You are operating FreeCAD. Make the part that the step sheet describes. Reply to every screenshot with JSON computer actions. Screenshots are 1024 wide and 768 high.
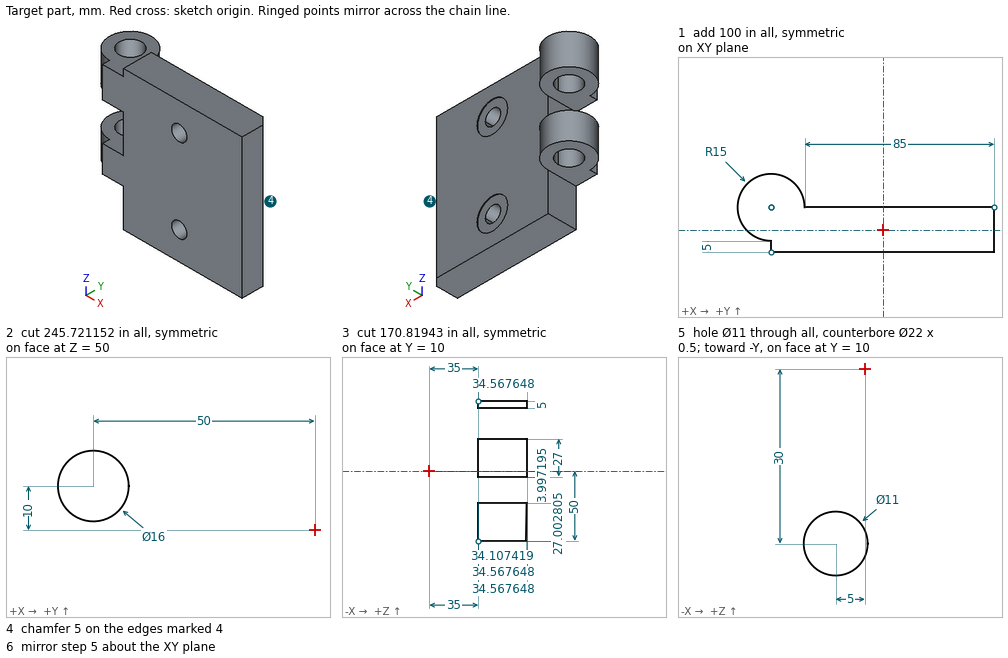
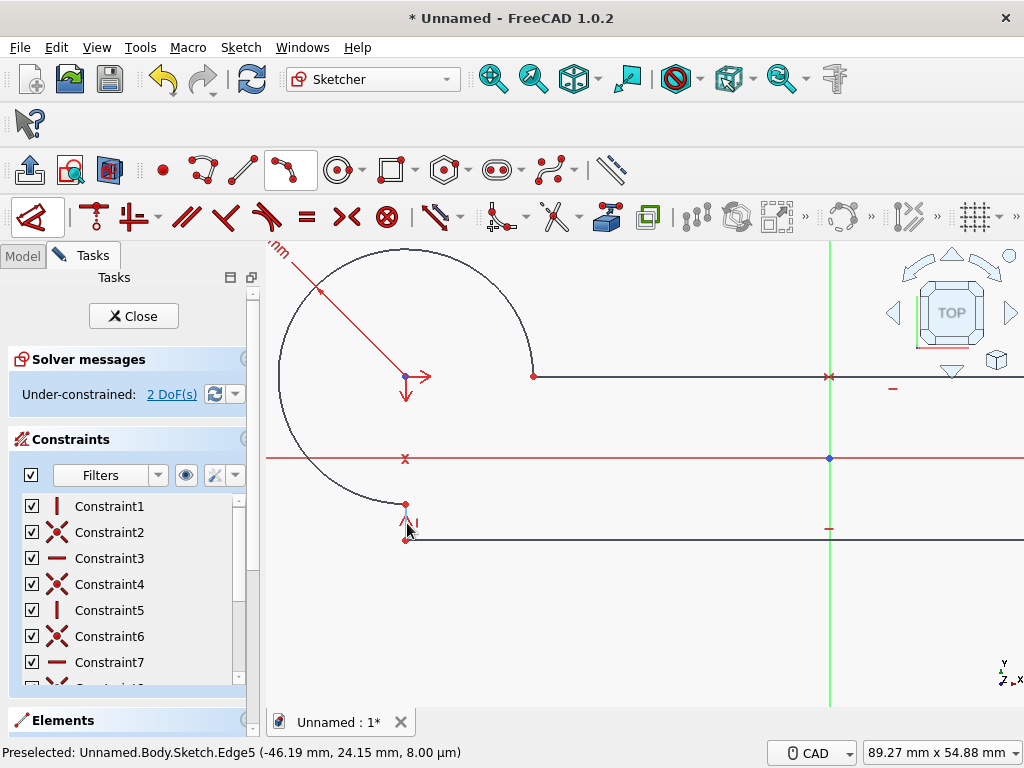
{"action": "left_click", "coordinate": [406, 522]}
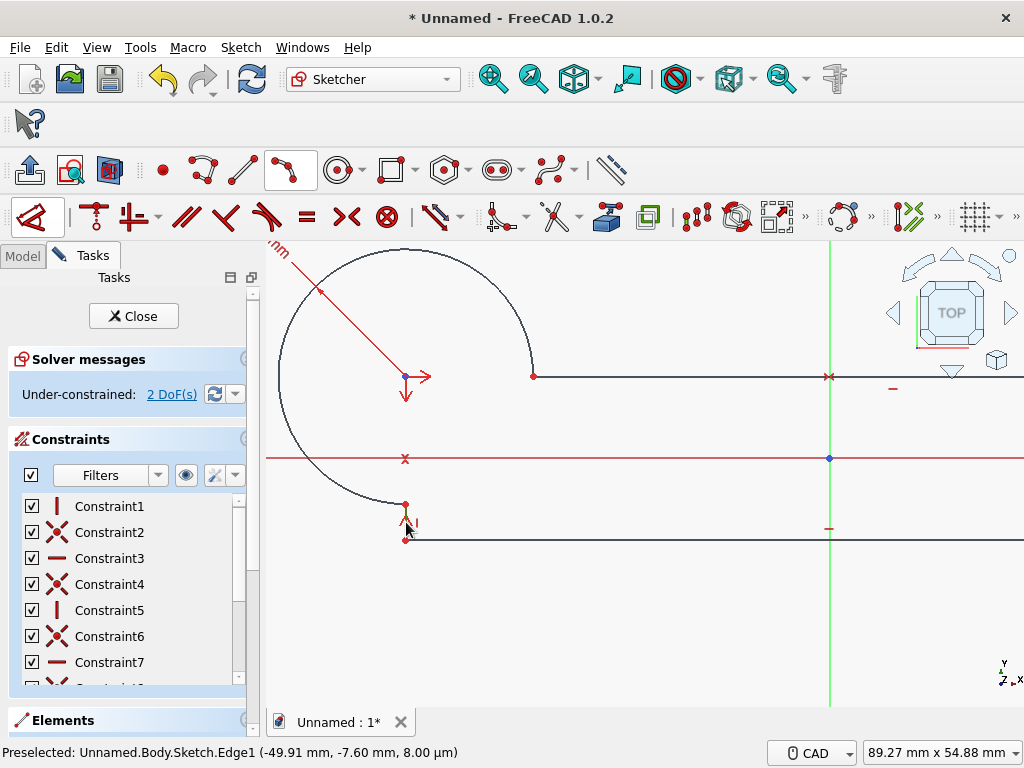
{"action": "left_click", "coordinate": [58, 218]}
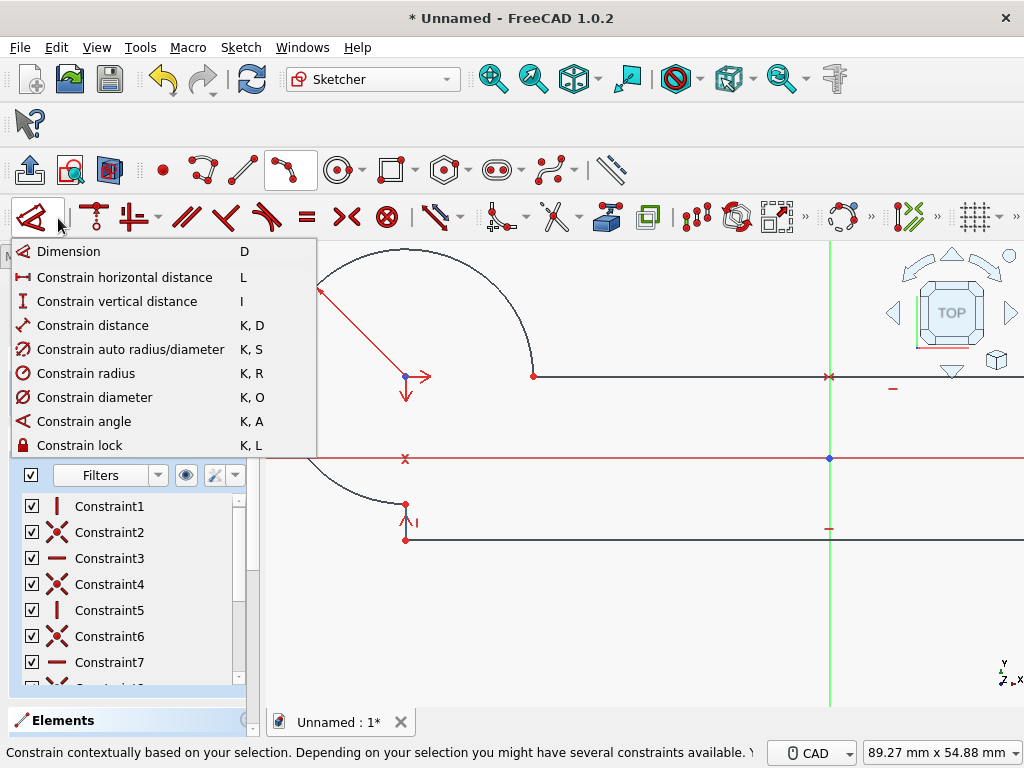
{"action": "left_click", "coordinate": [164, 301]}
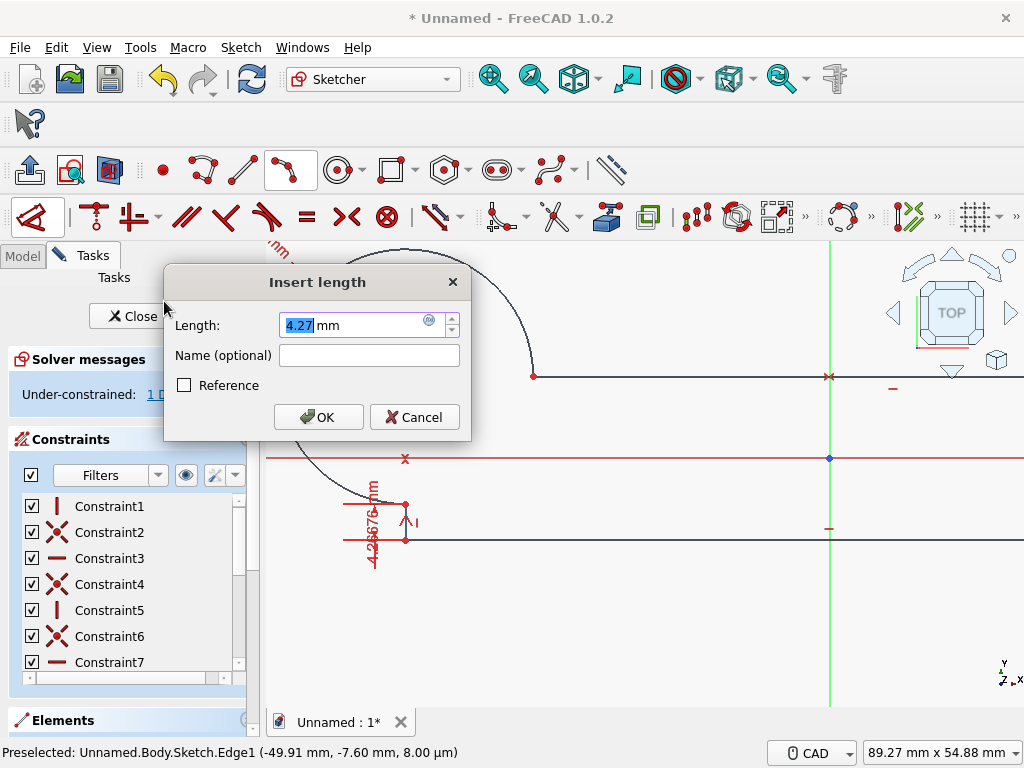
{"action": "type", "text": "5"}
{"action": "key", "text": "Return"}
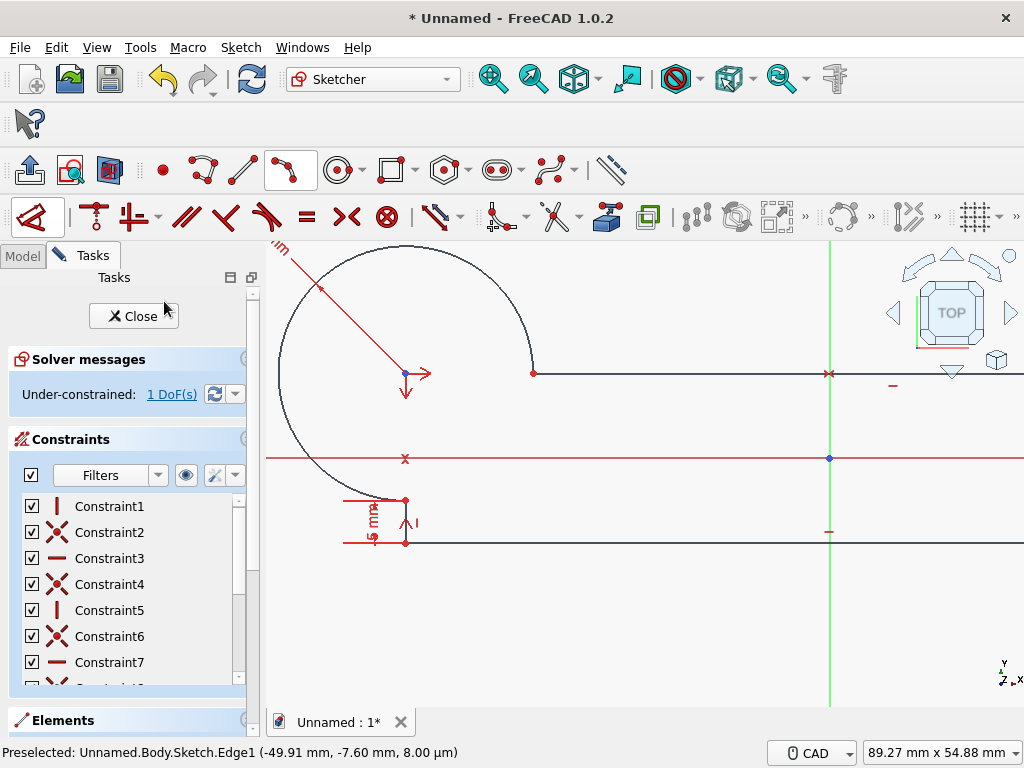
{"action": "left_click", "coordinate": [749, 374]}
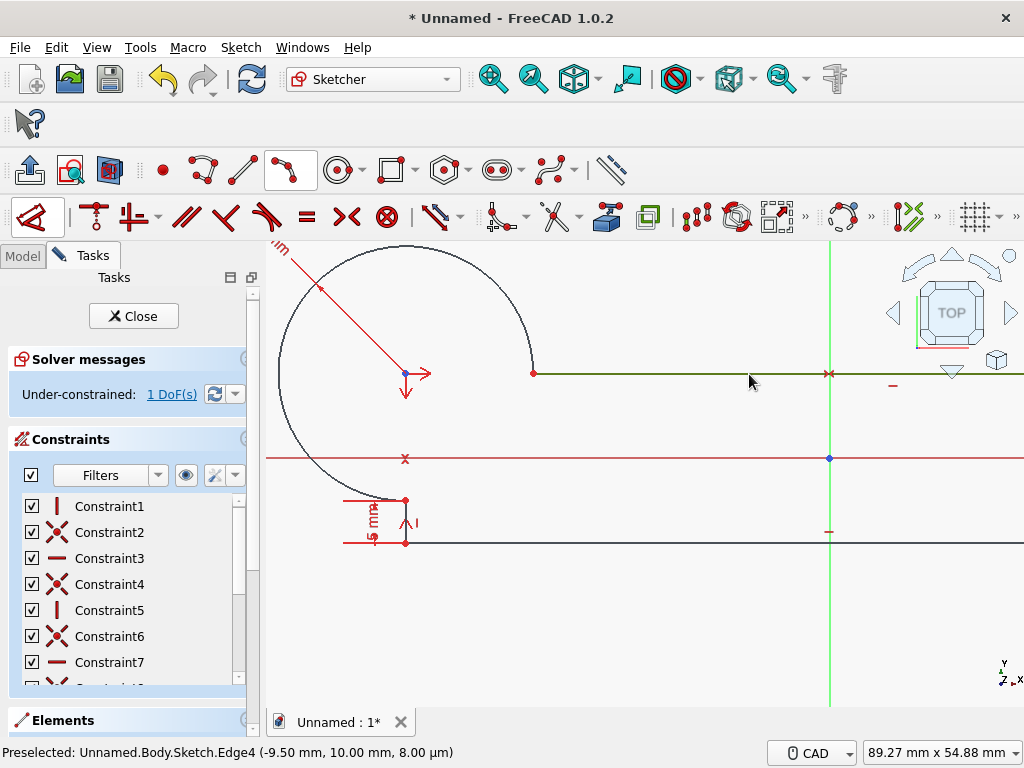
{"action": "key", "text": "l"}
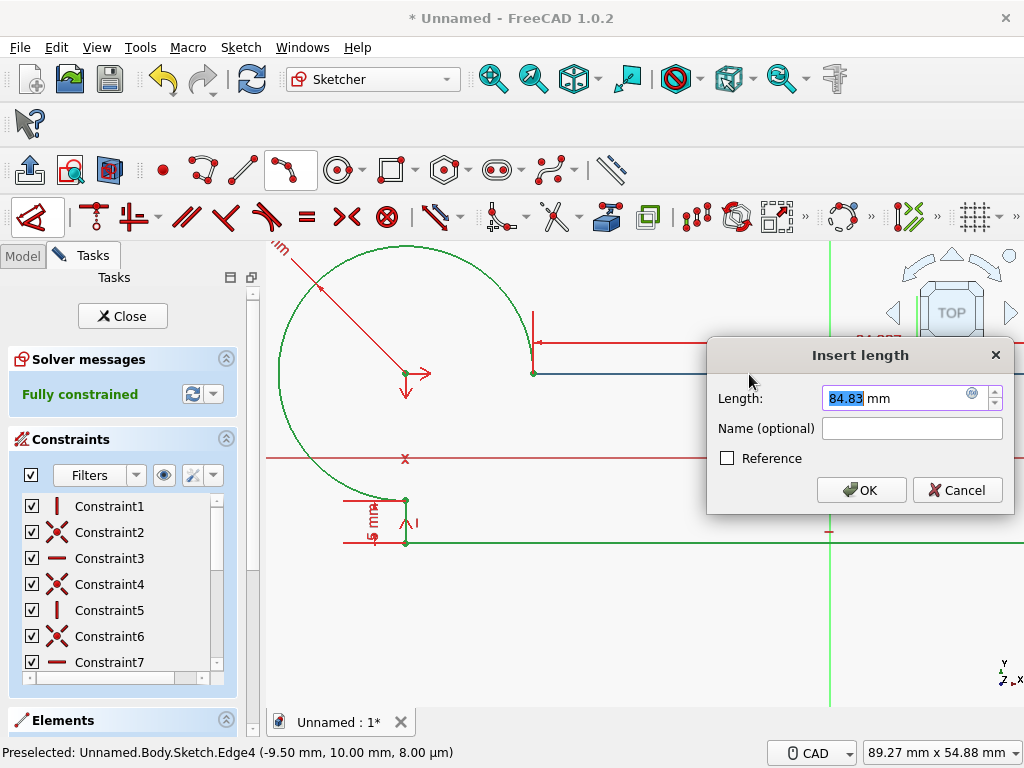
{"action": "type", "text": "85"}
{"action": "key", "text": "Return"}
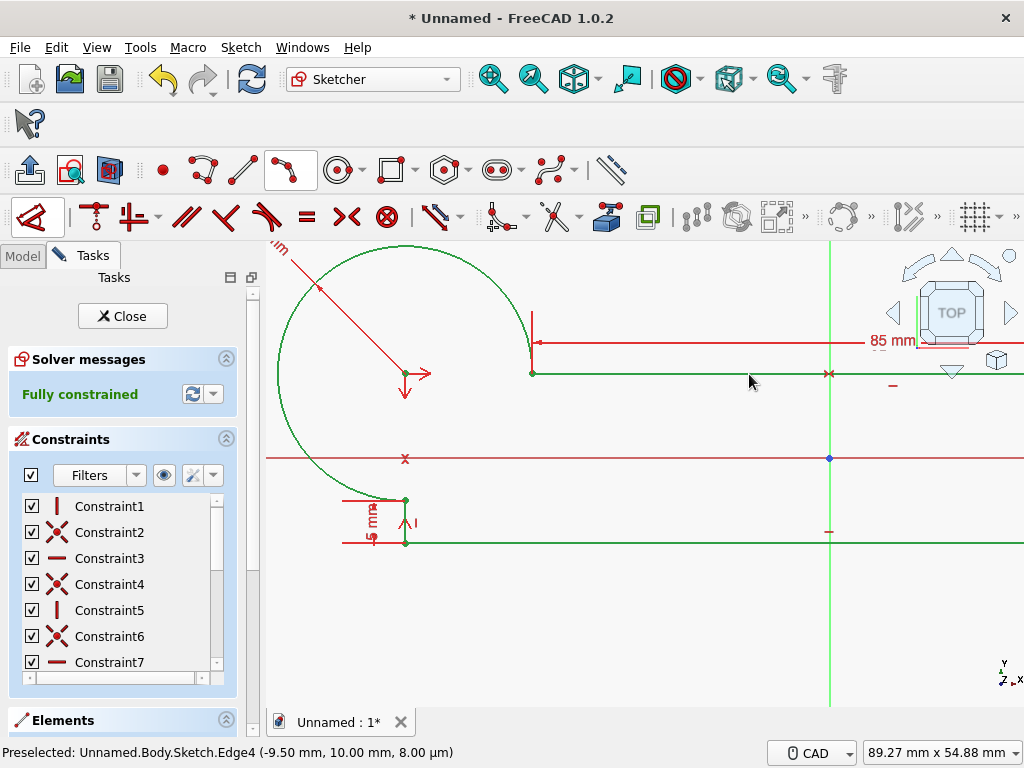
{"action": "left_click", "coordinate": [123, 316]}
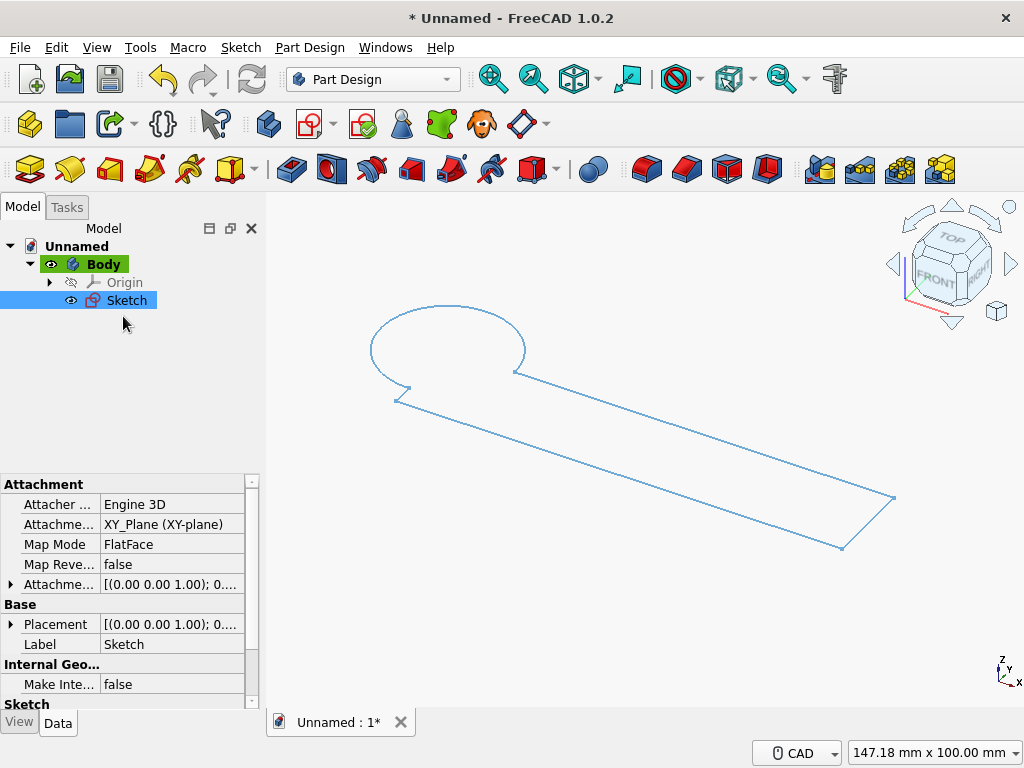
{"action": "left_click", "coordinate": [30, 170]}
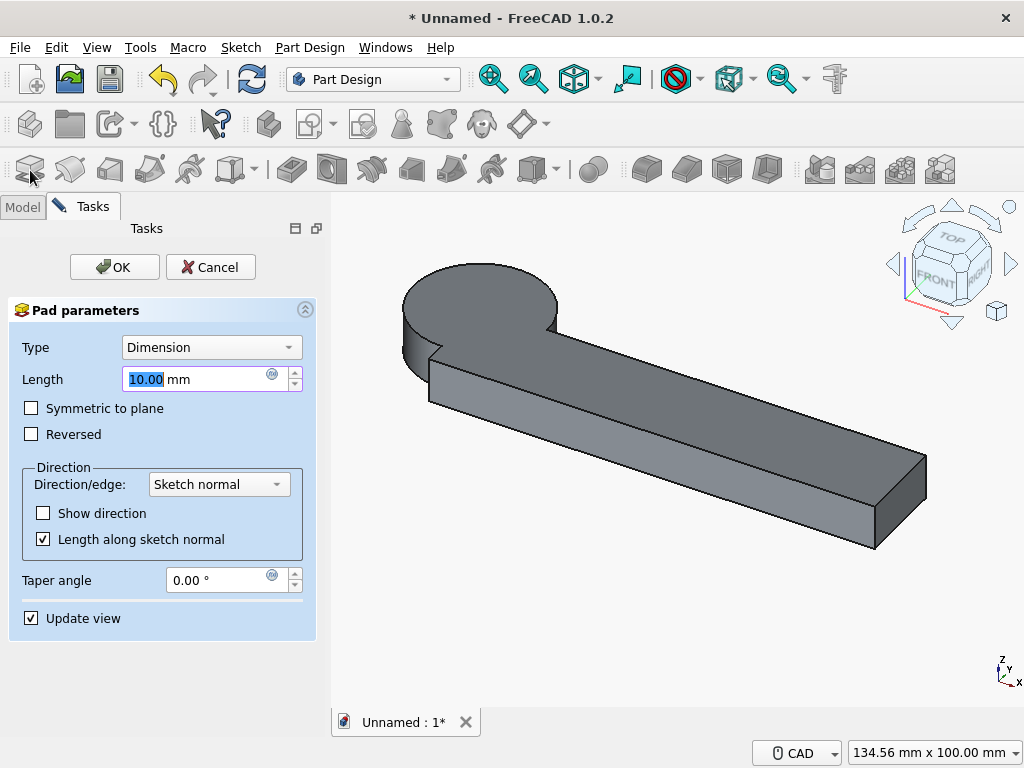
{"action": "type", "text": "100"}
{"action": "key", "text": "Tab"}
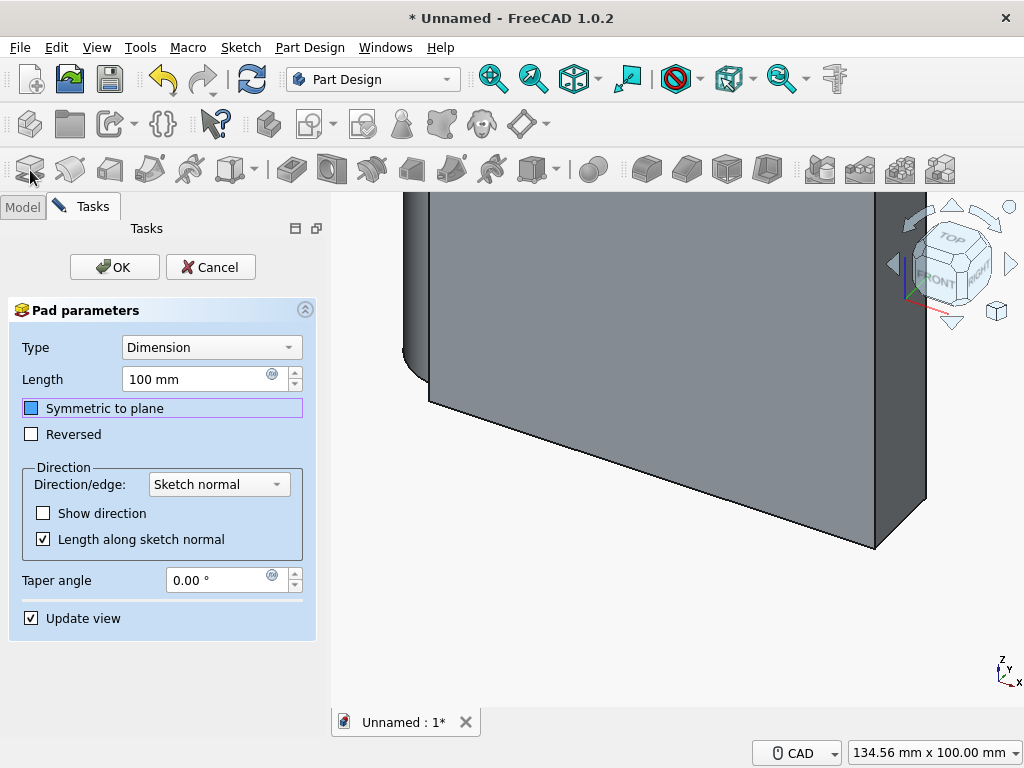
{"action": "left_click", "coordinate": [30, 408]}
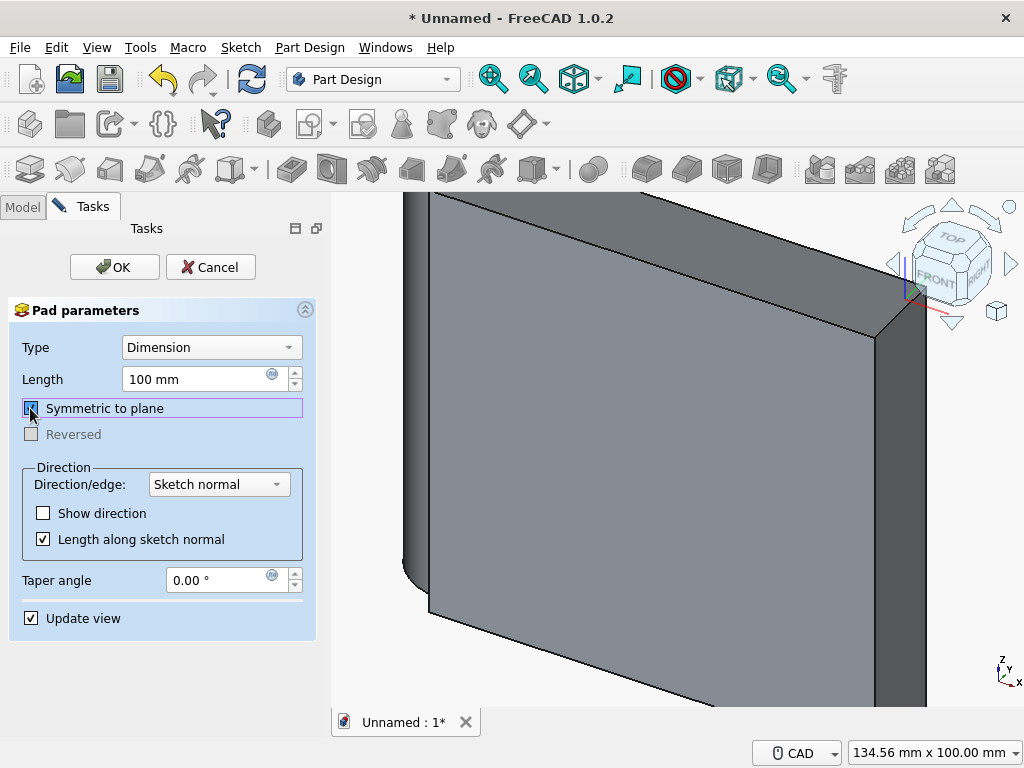
{"action": "left_click", "coordinate": [115, 267]}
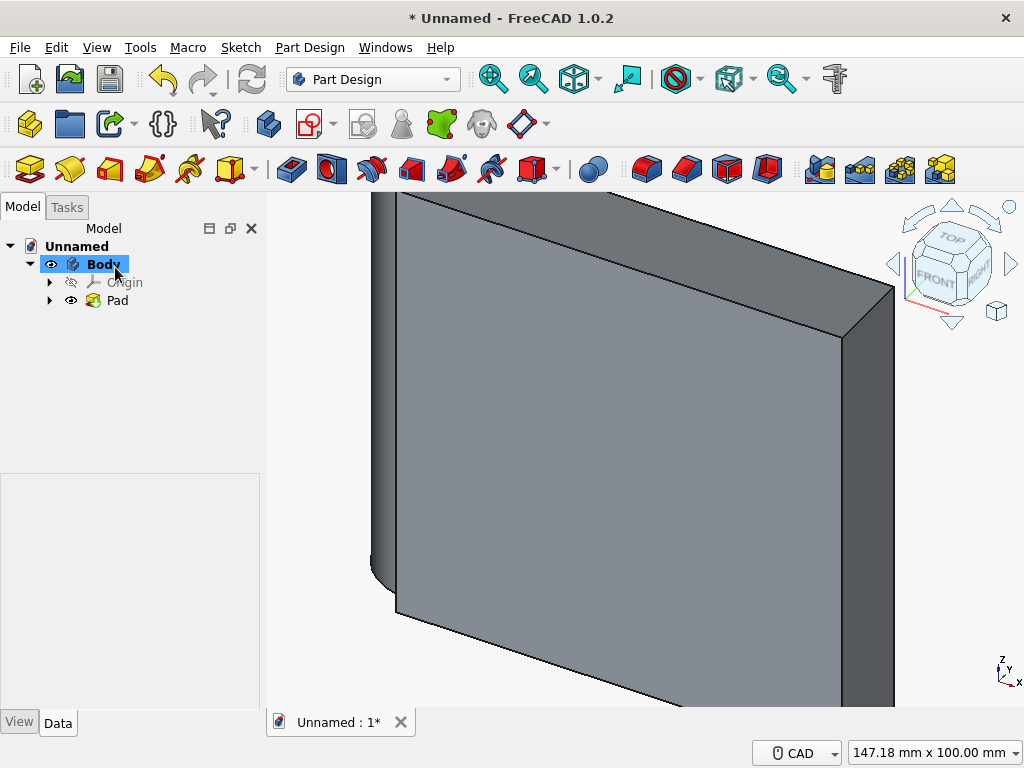
{"action": "left_click", "coordinate": [494, 80]}